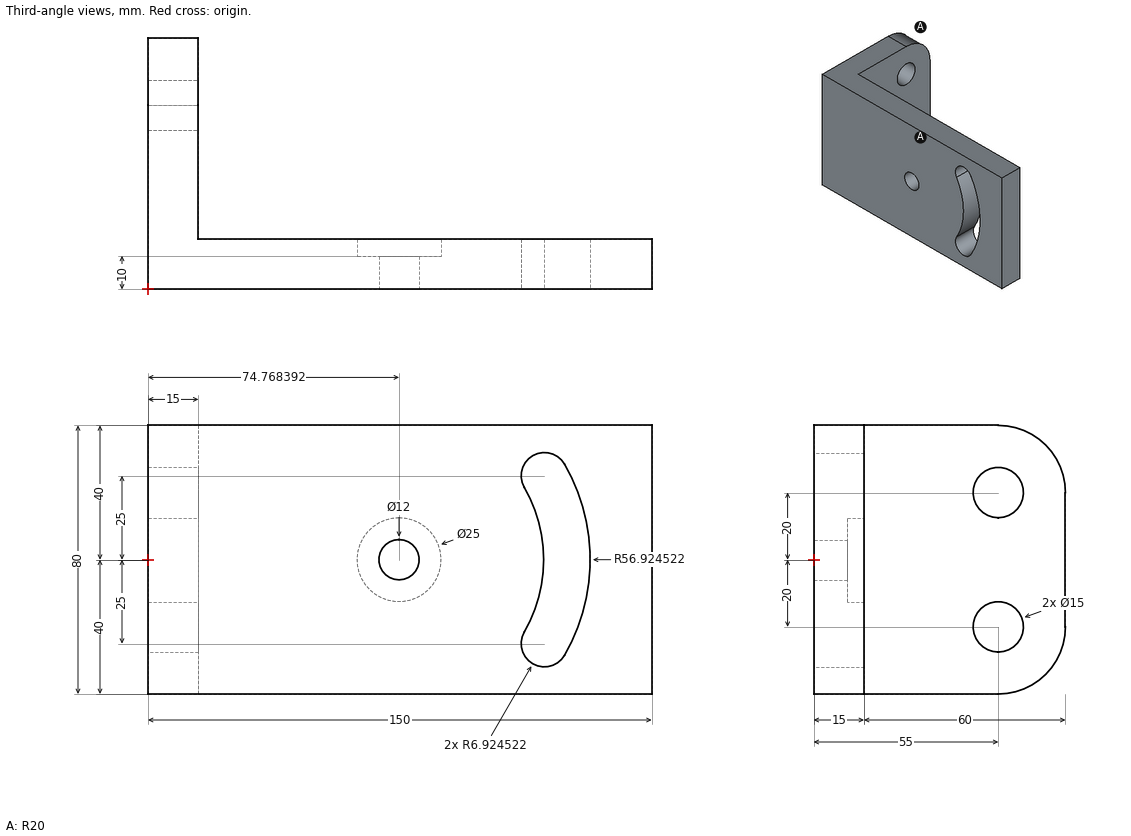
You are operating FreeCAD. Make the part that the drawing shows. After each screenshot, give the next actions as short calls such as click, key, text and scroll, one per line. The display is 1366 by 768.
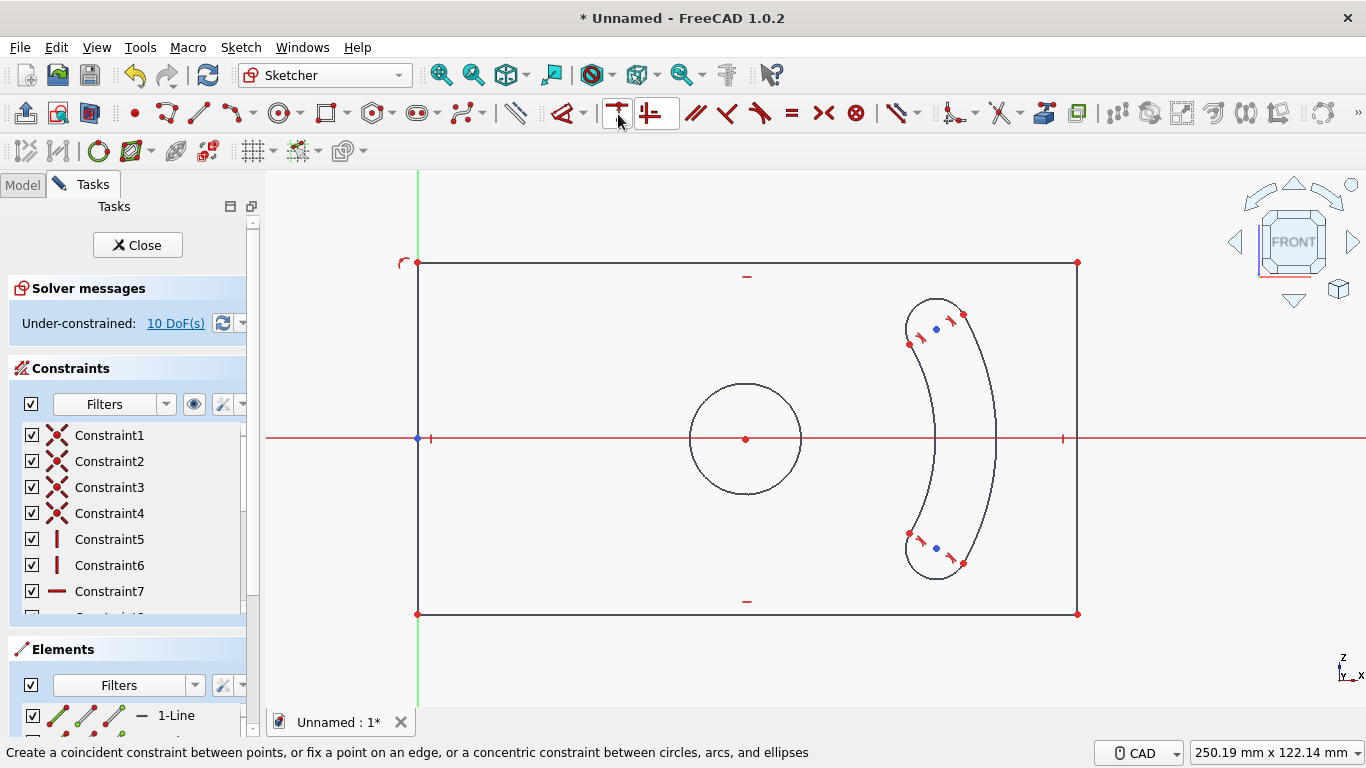
click(745, 439)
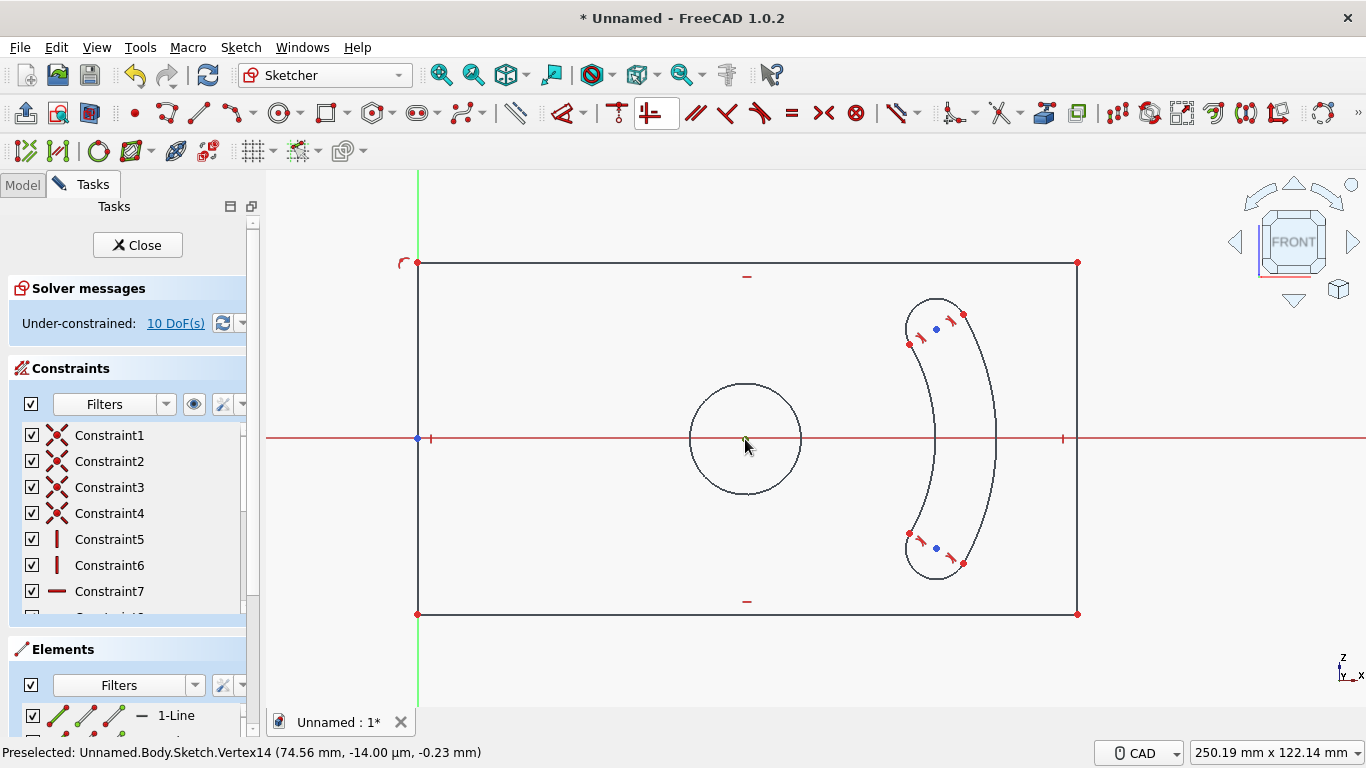
click(359, 438)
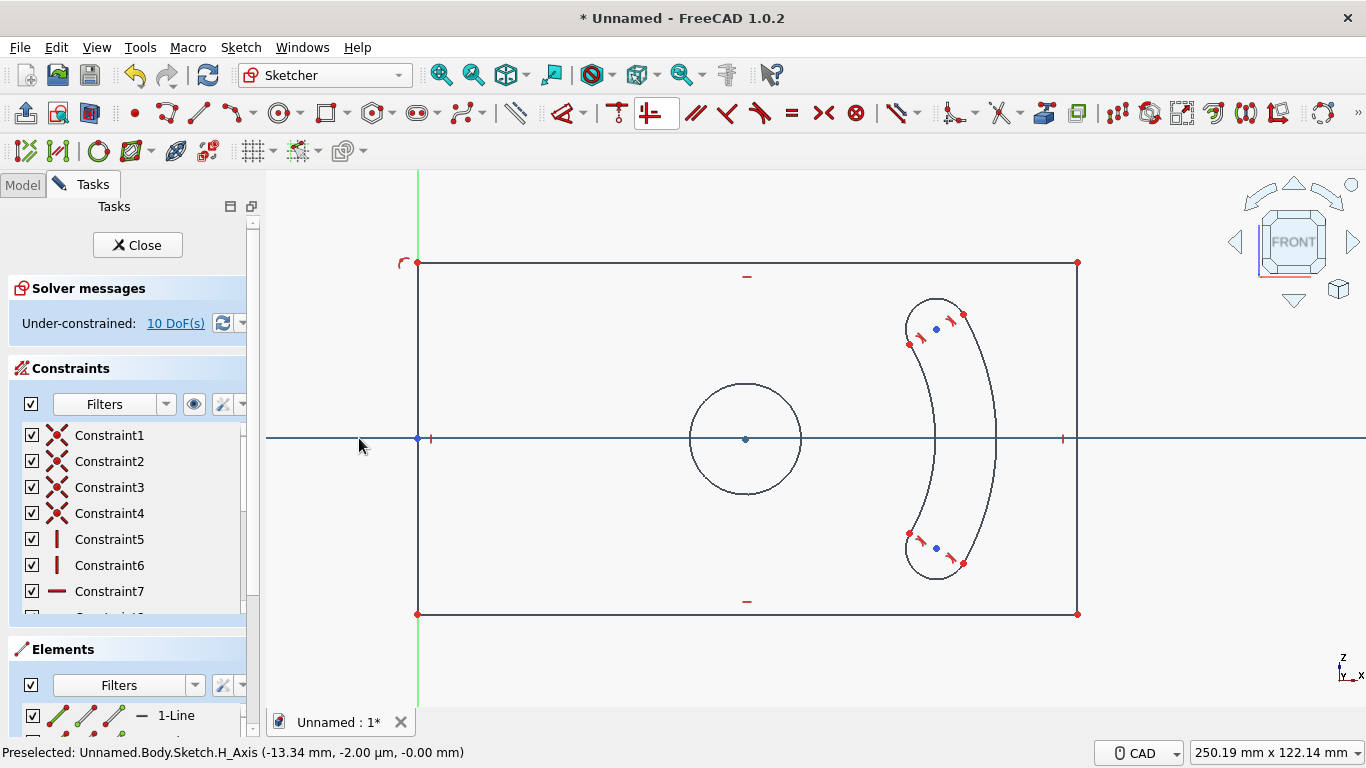
click(618, 114)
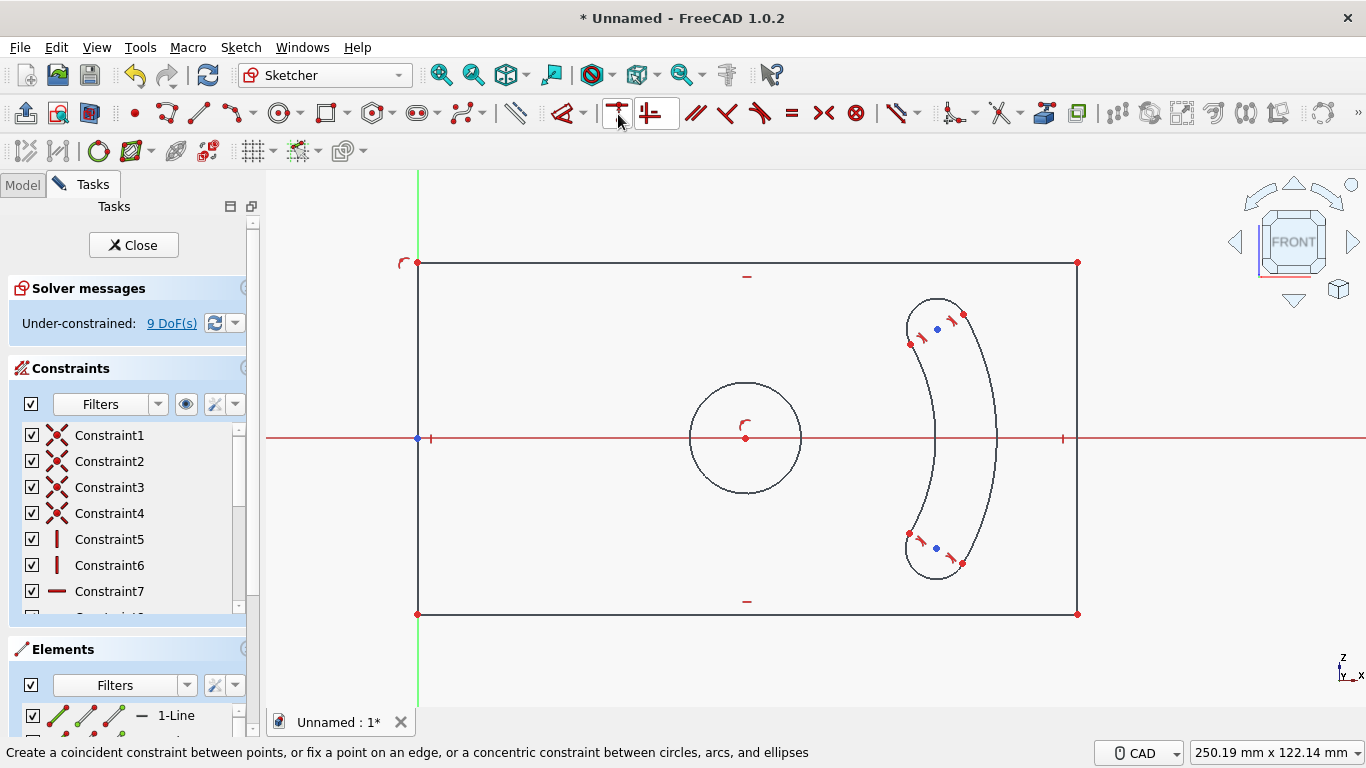
key(d)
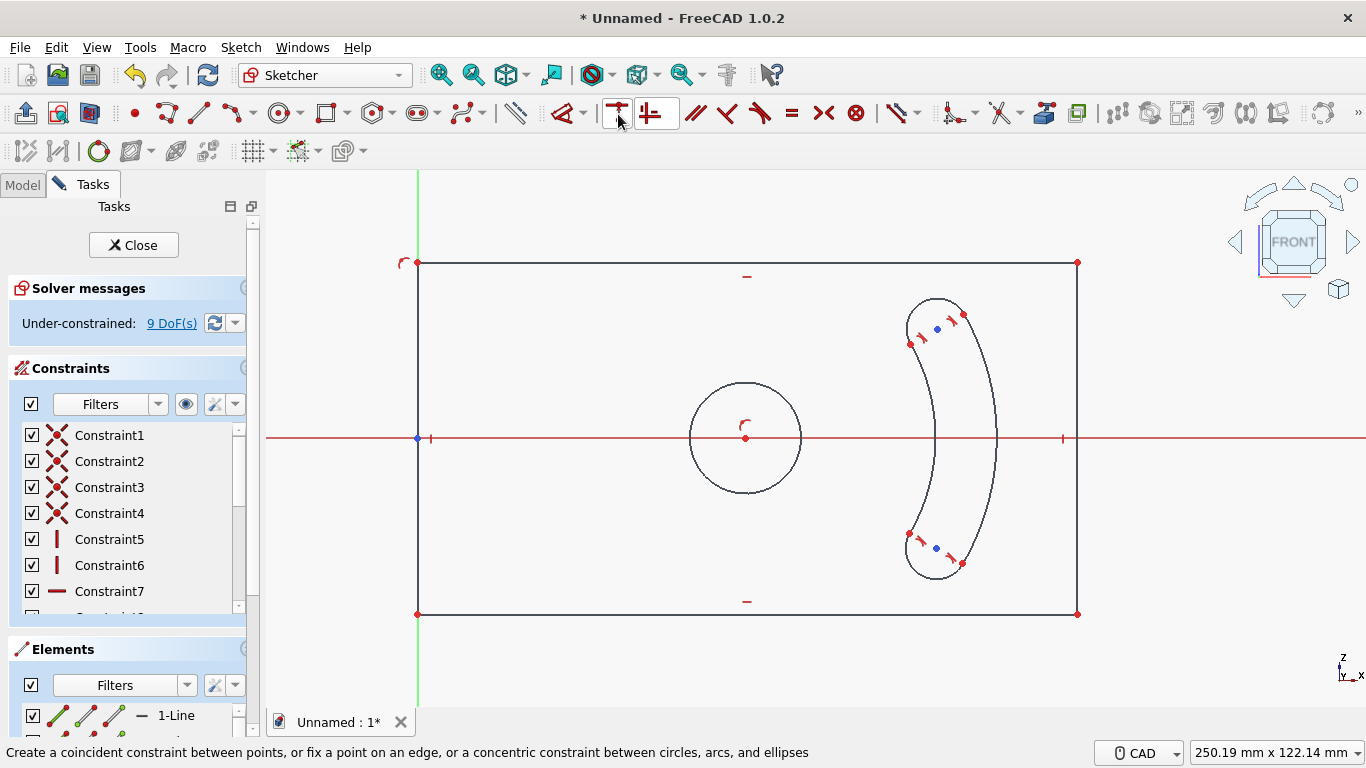
scroll(908, 561, up, 2)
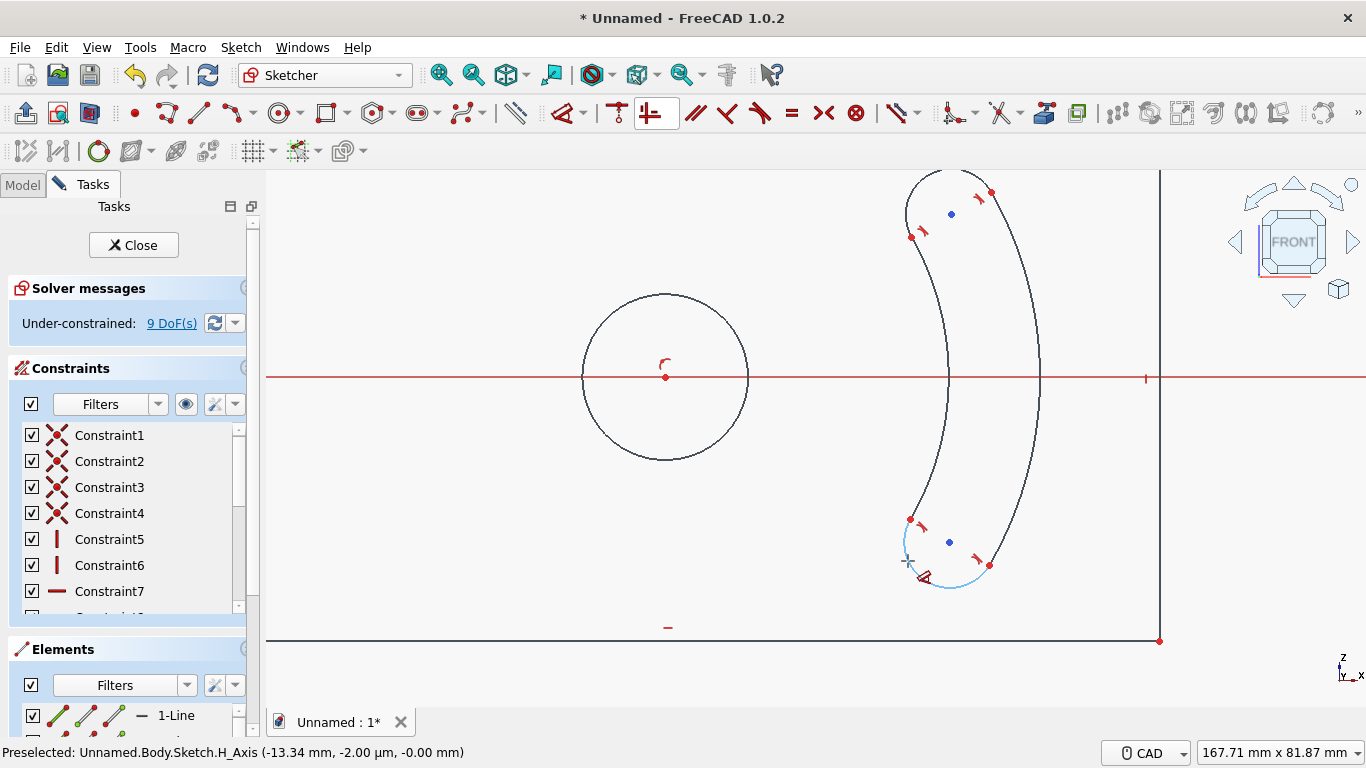
click(908, 561)
click(879, 574)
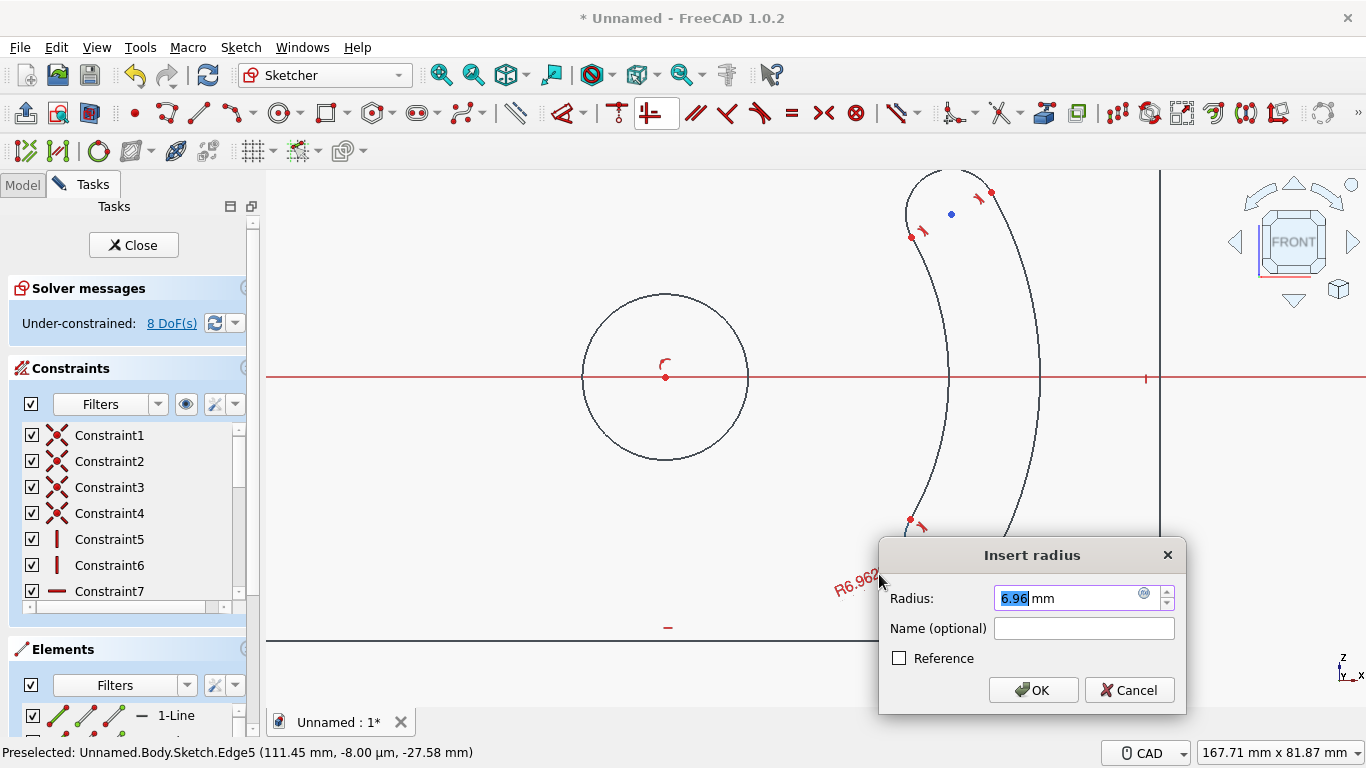
text(6.924522)
key(Return)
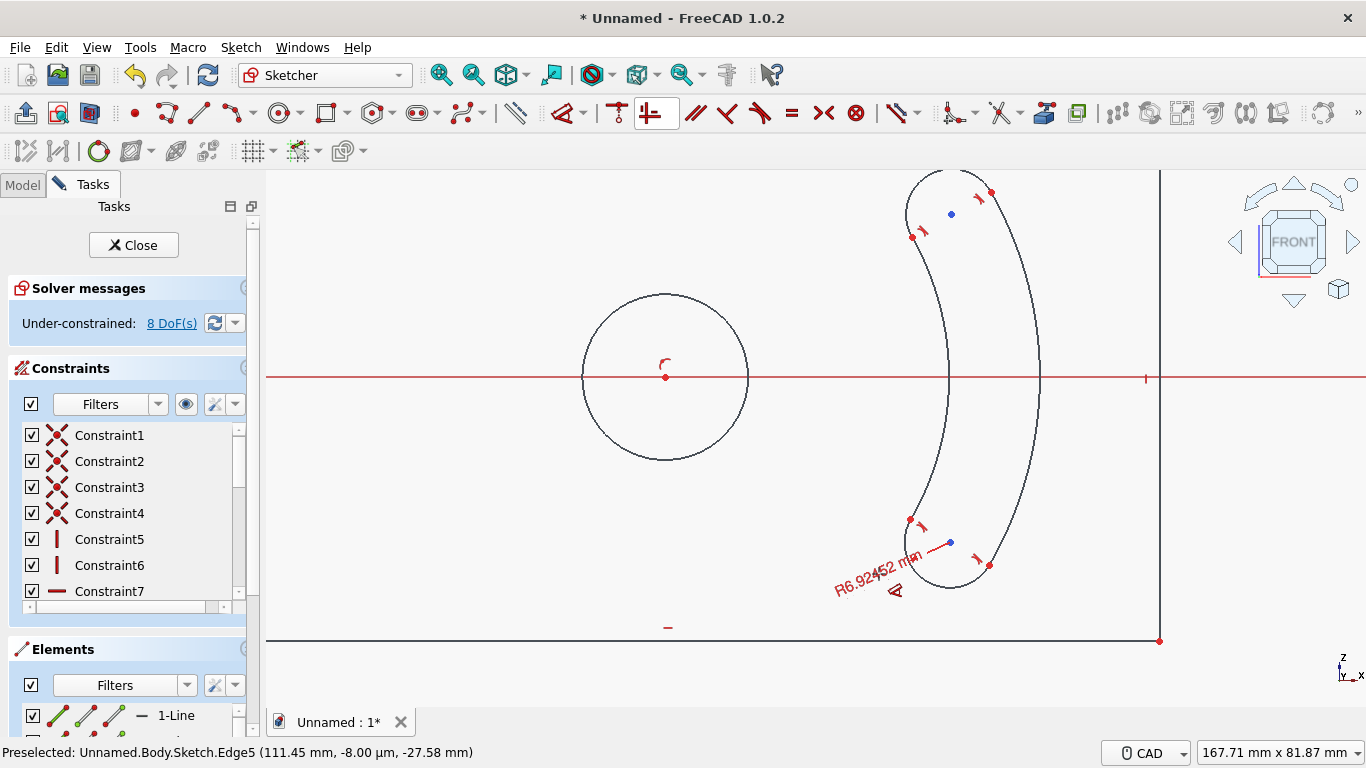
click(1031, 456)
click(1062, 463)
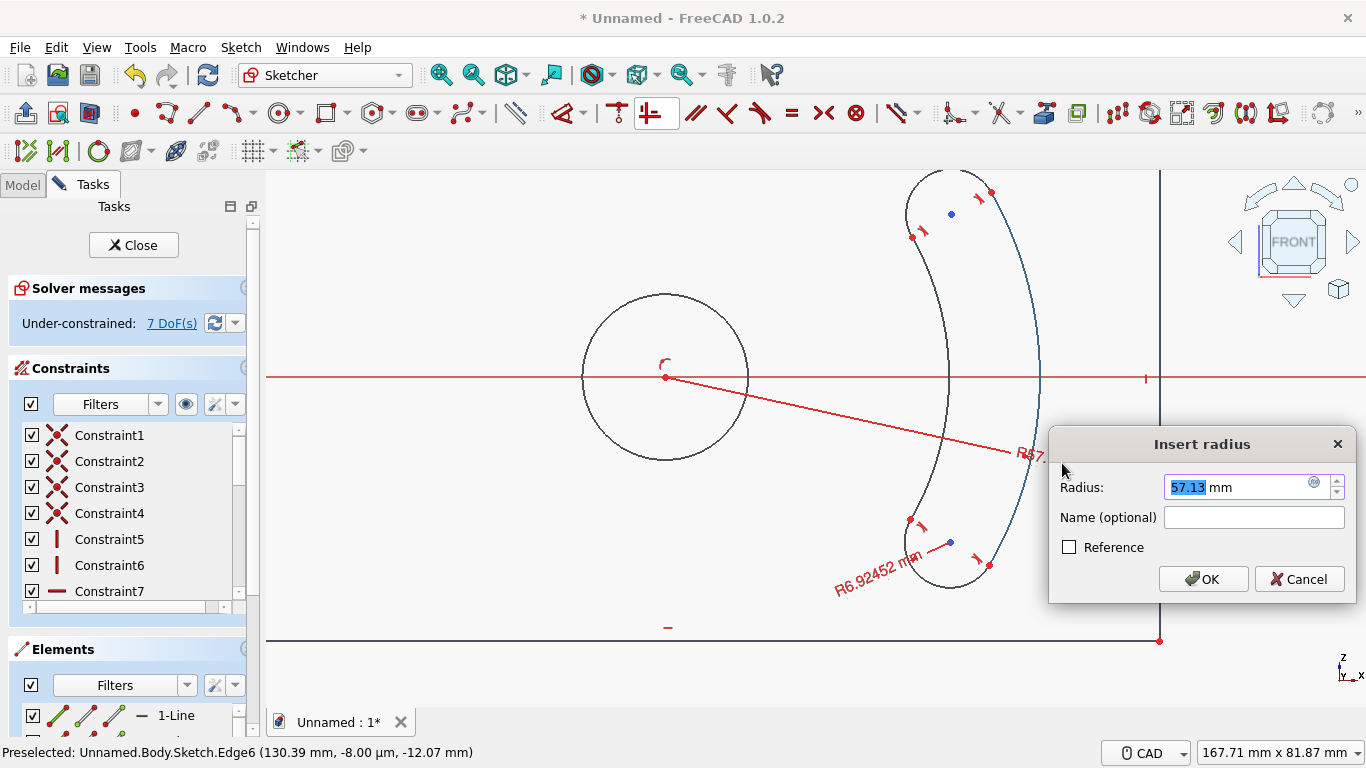
text(56.924522)
key(Return)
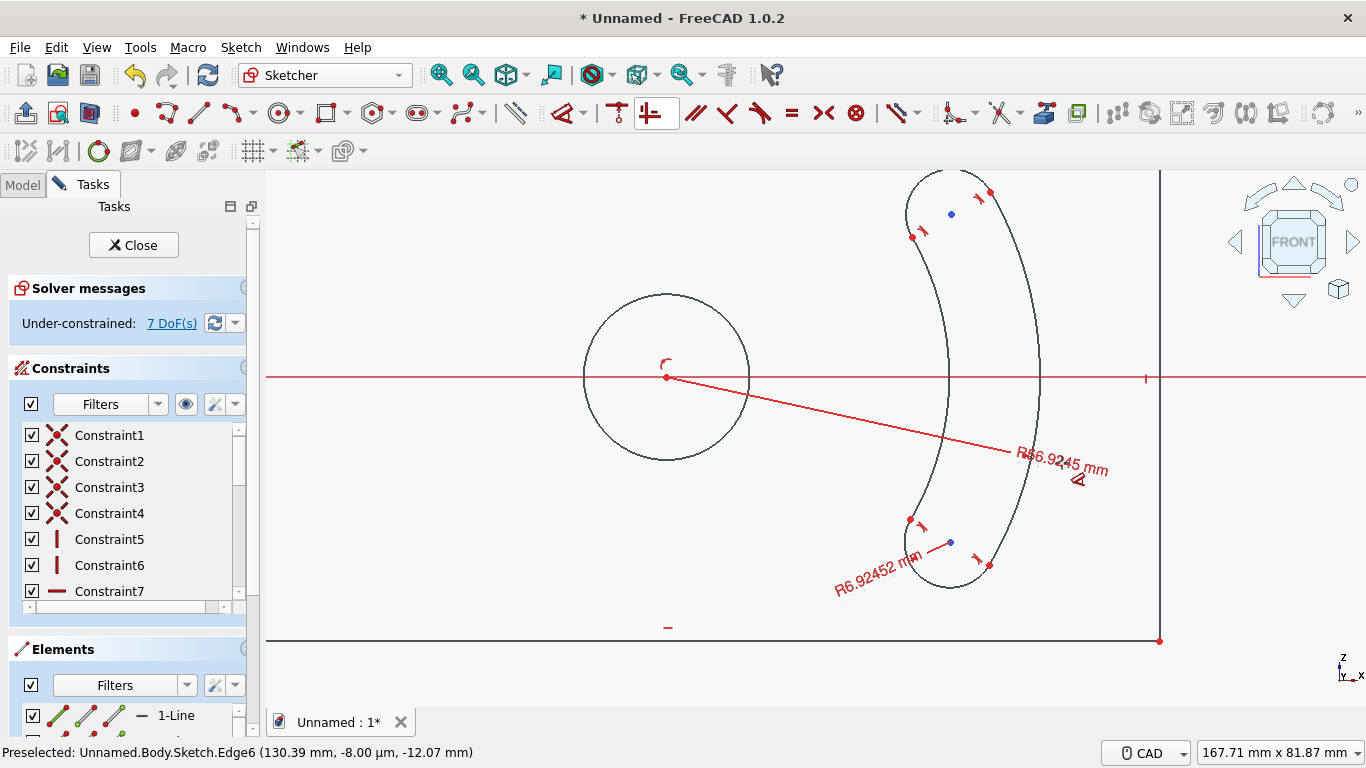
click(725, 318)
click(747, 295)